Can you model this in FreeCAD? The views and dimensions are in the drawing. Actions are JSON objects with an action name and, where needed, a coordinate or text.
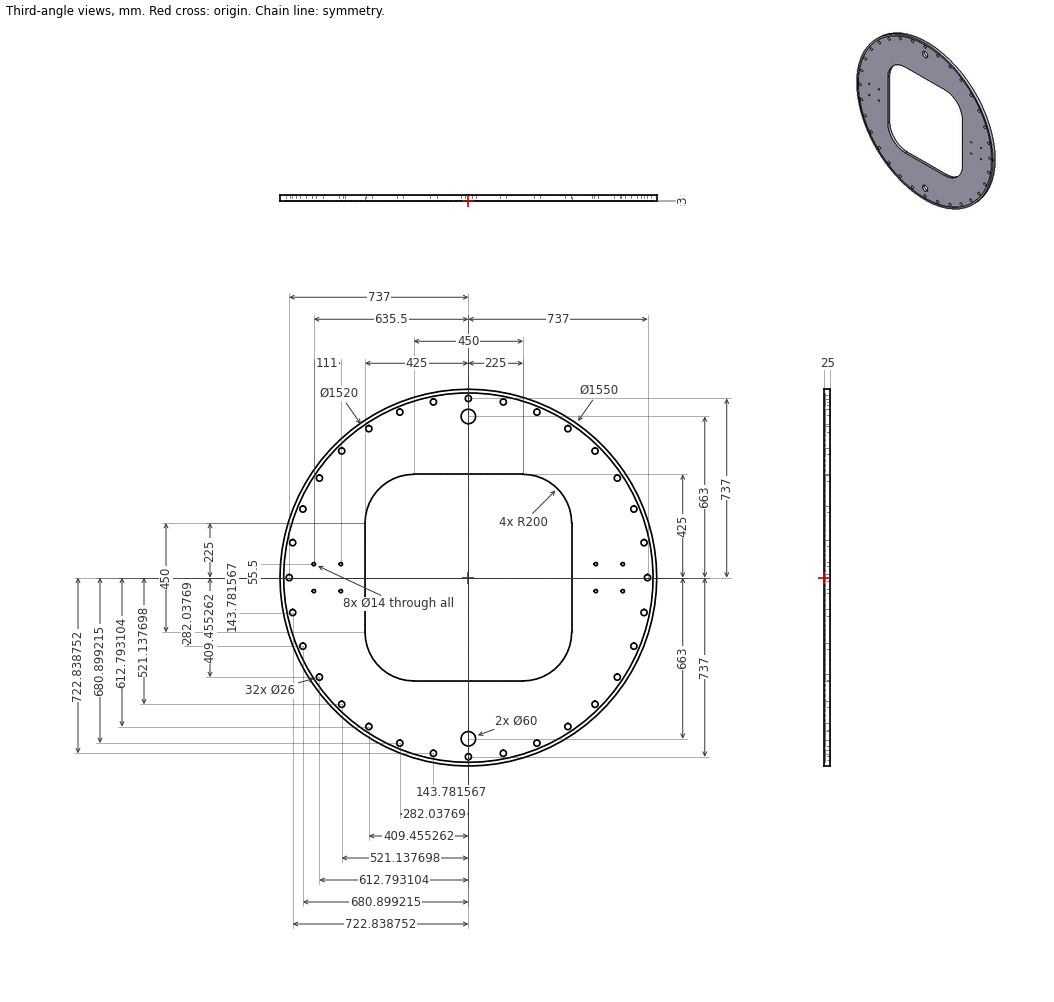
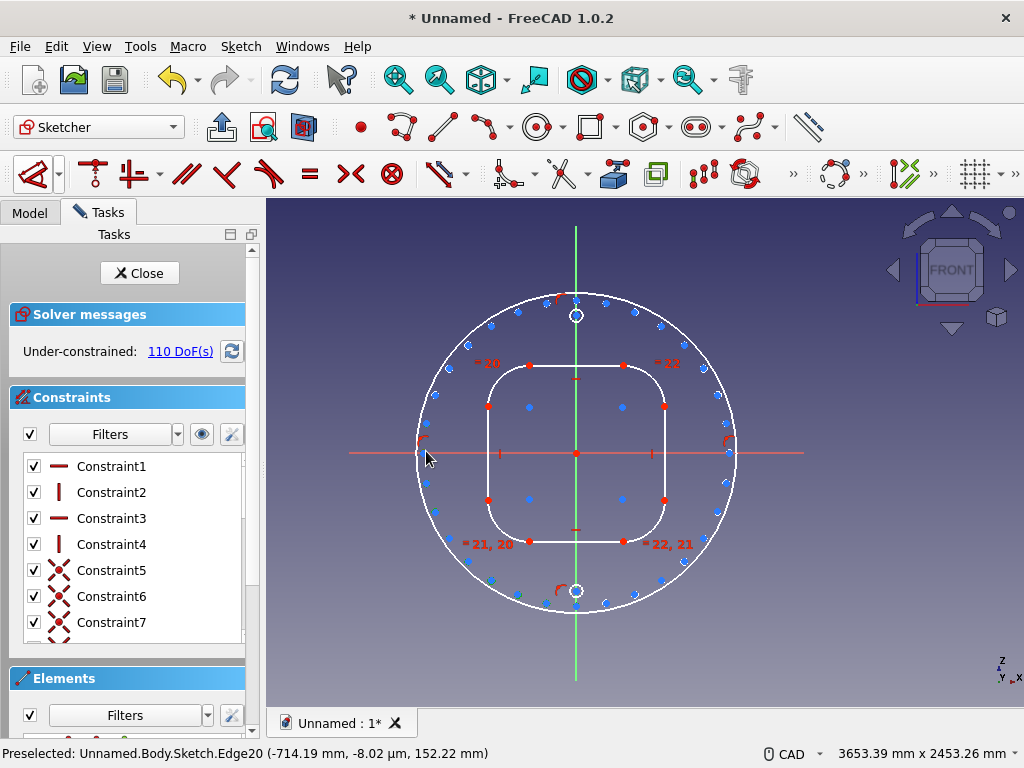
{"action": "scroll", "coordinate": [437, 393], "scroll_direction": "up", "scroll_amount": 8}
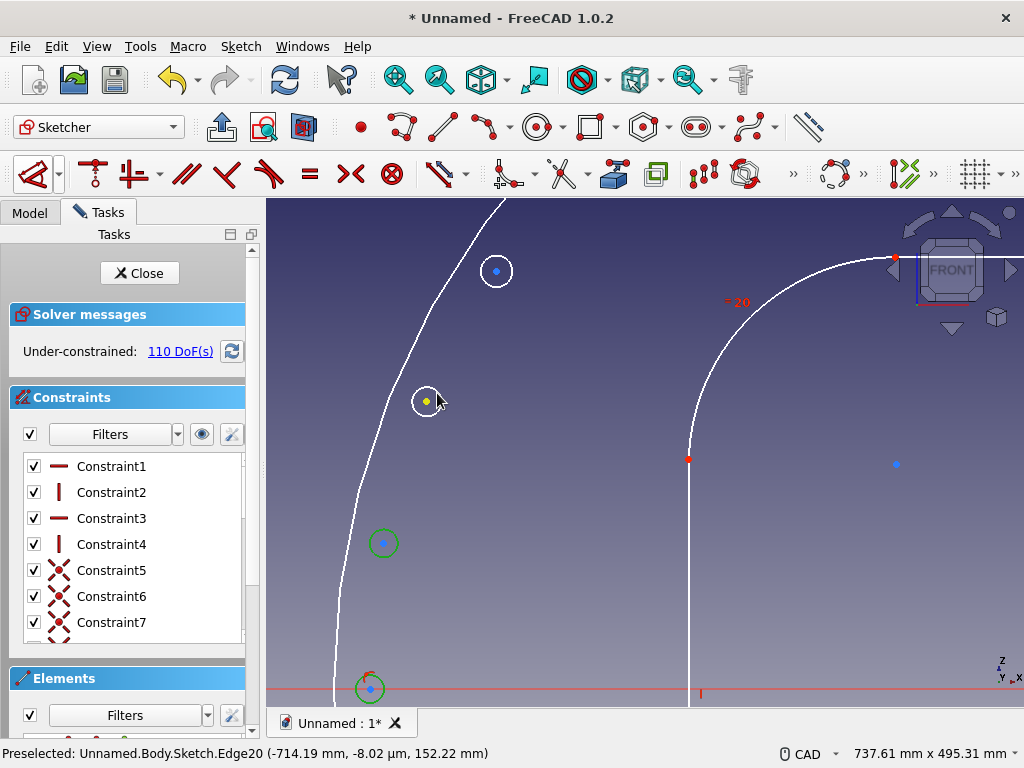
{"action": "left_click", "coordinate": [437, 391]}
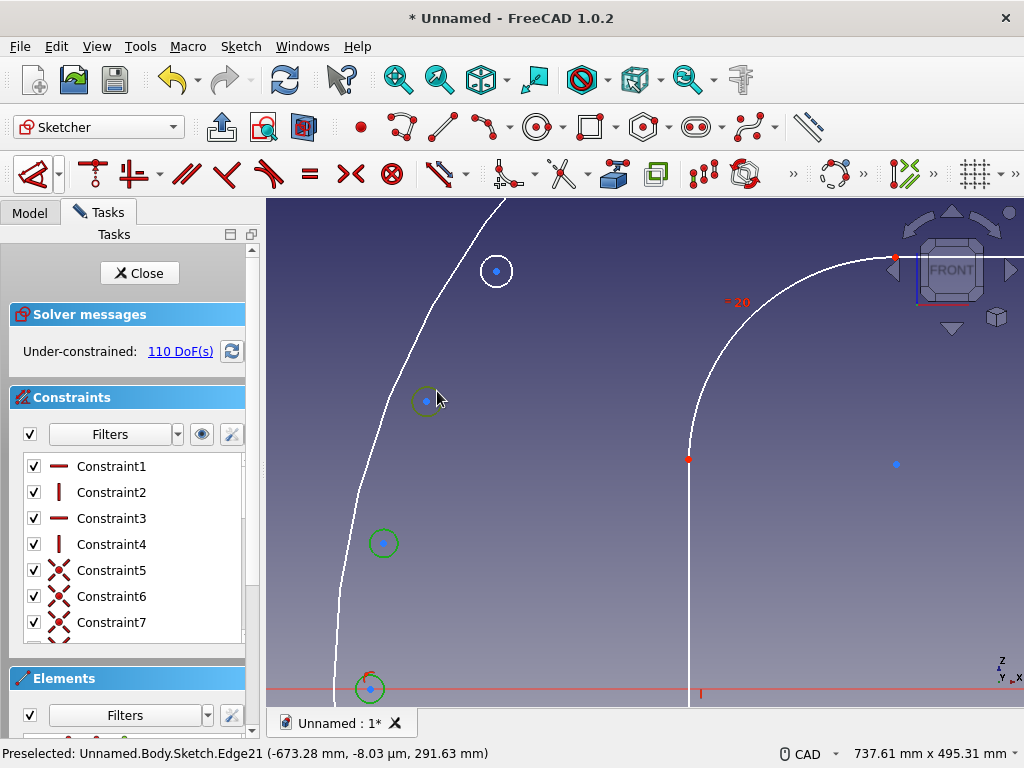
{"action": "left_click", "coordinate": [508, 260]}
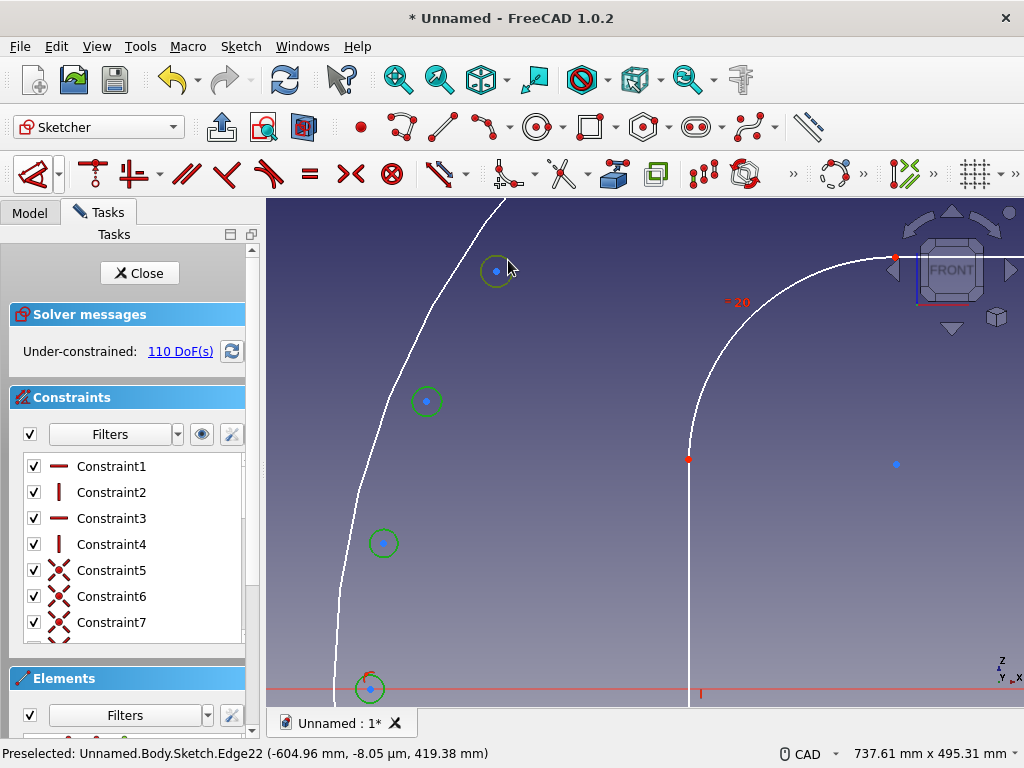
{"action": "scroll", "coordinate": [437, 393], "scroll_direction": "down", "scroll_amount": 8}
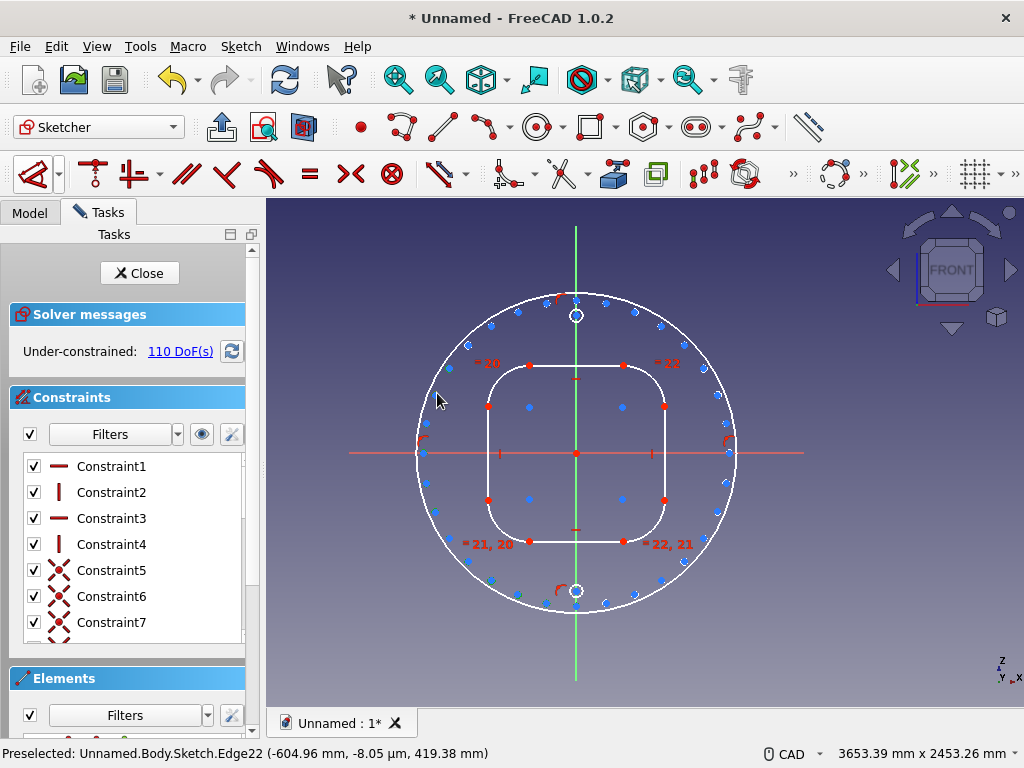
{"action": "scroll", "coordinate": [470, 343], "scroll_direction": "up", "scroll_amount": 8}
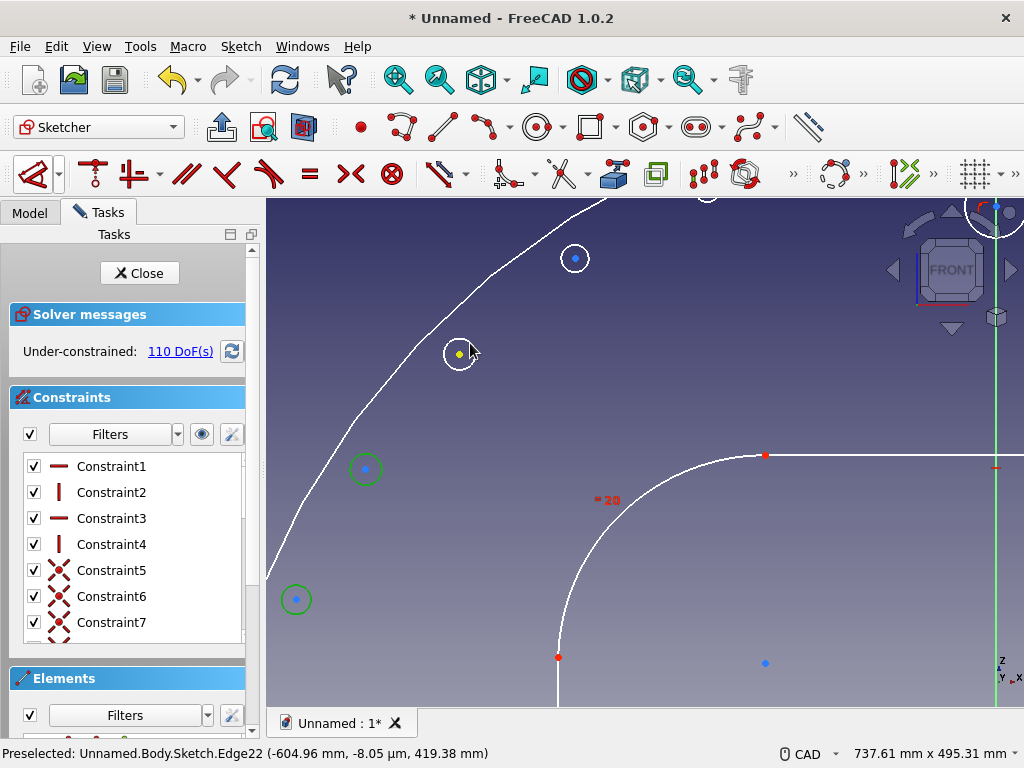
{"action": "left_click", "coordinate": [471, 343]}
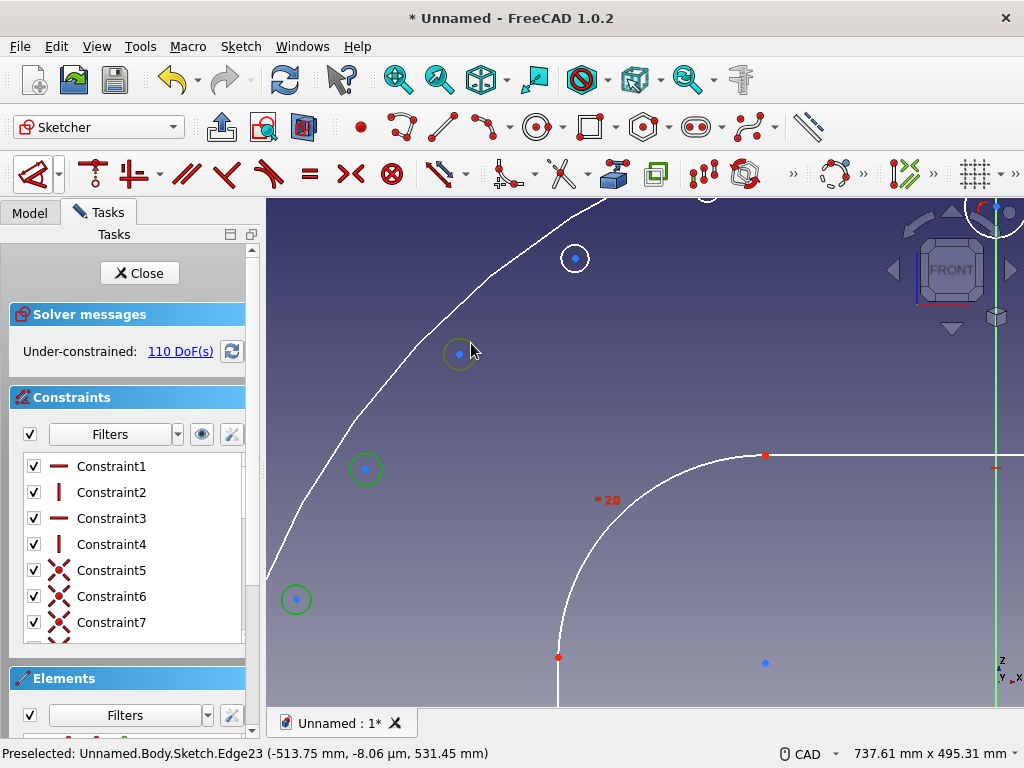
{"action": "left_click", "coordinate": [585, 249]}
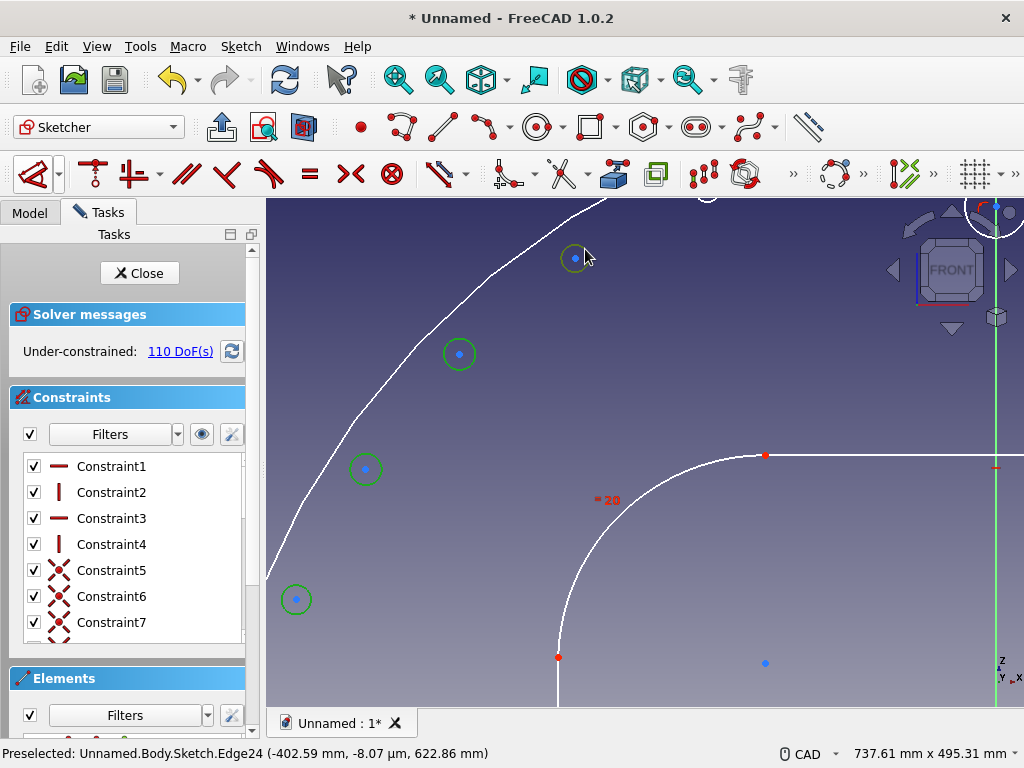
{"action": "scroll", "coordinate": [470, 343], "scroll_direction": "down", "scroll_amount": 8}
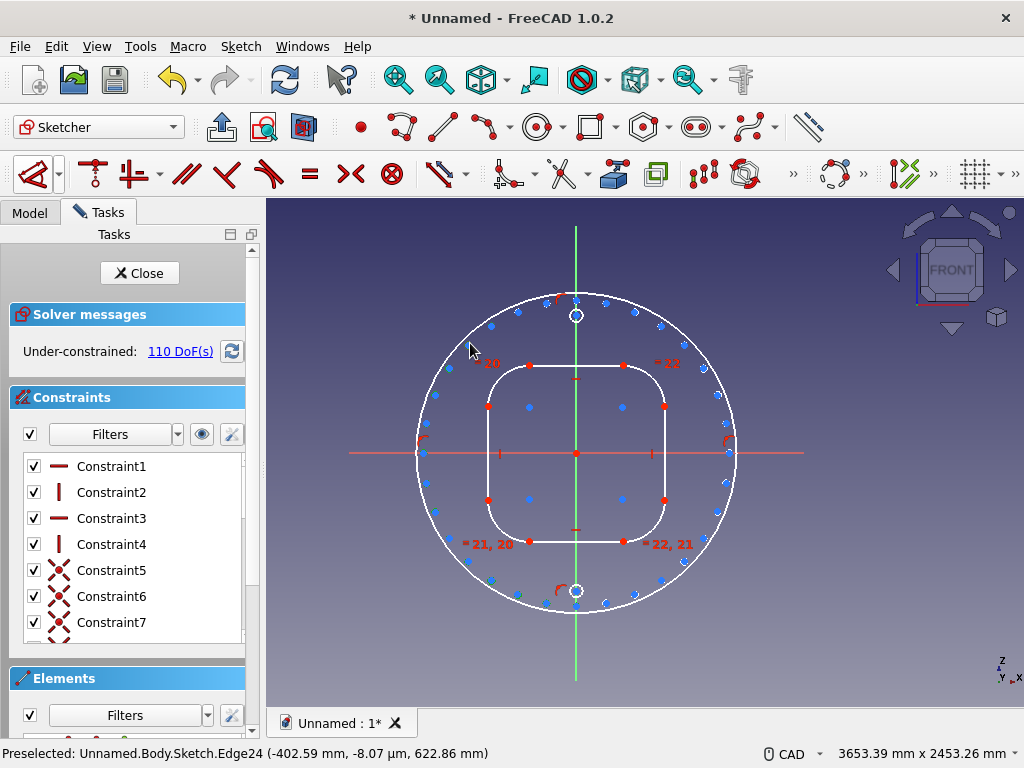
{"action": "scroll", "coordinate": [520, 310], "scroll_direction": "up", "scroll_amount": 9}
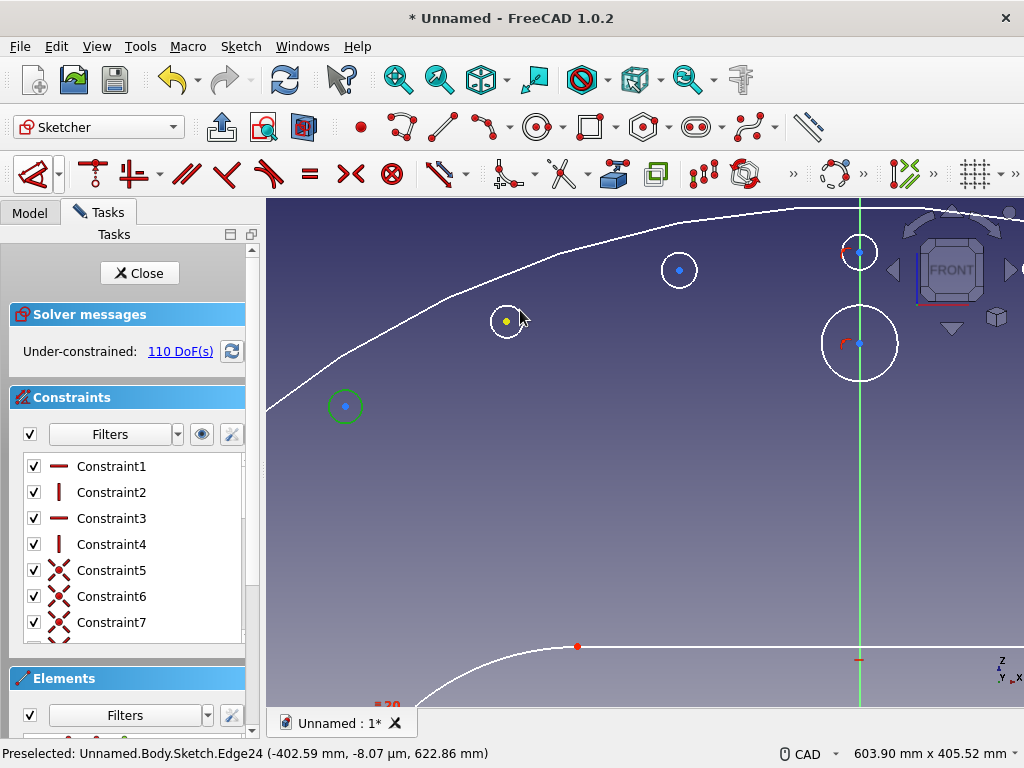
{"action": "left_click", "coordinate": [518, 310]}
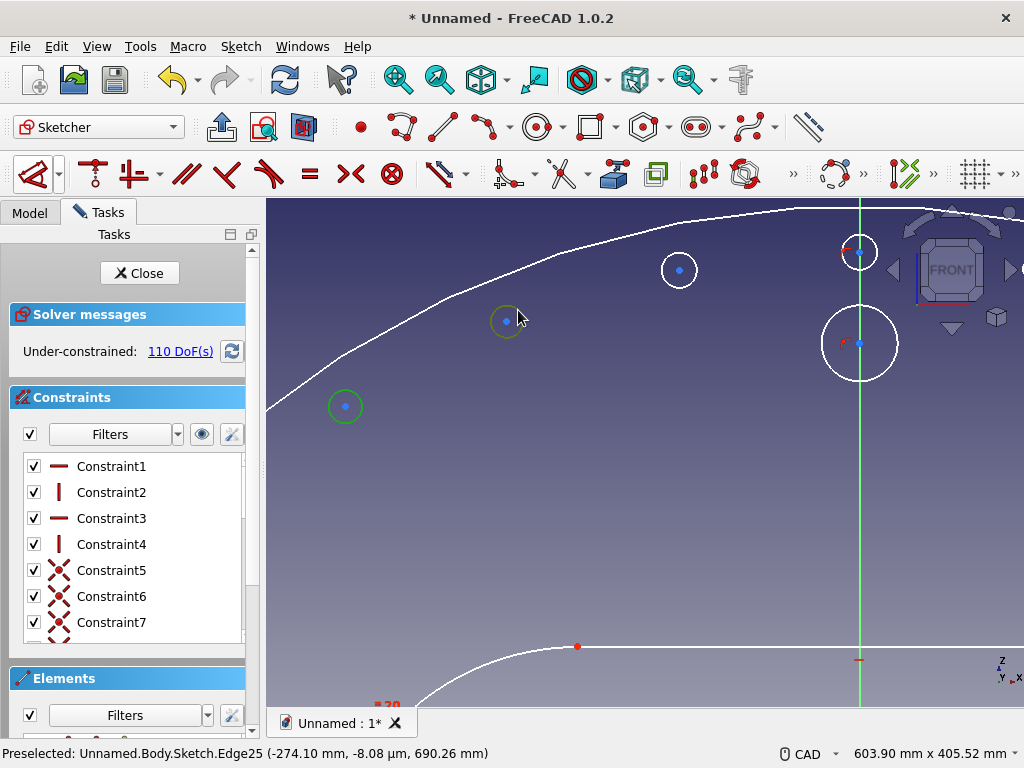
{"action": "left_click", "coordinate": [692, 258]}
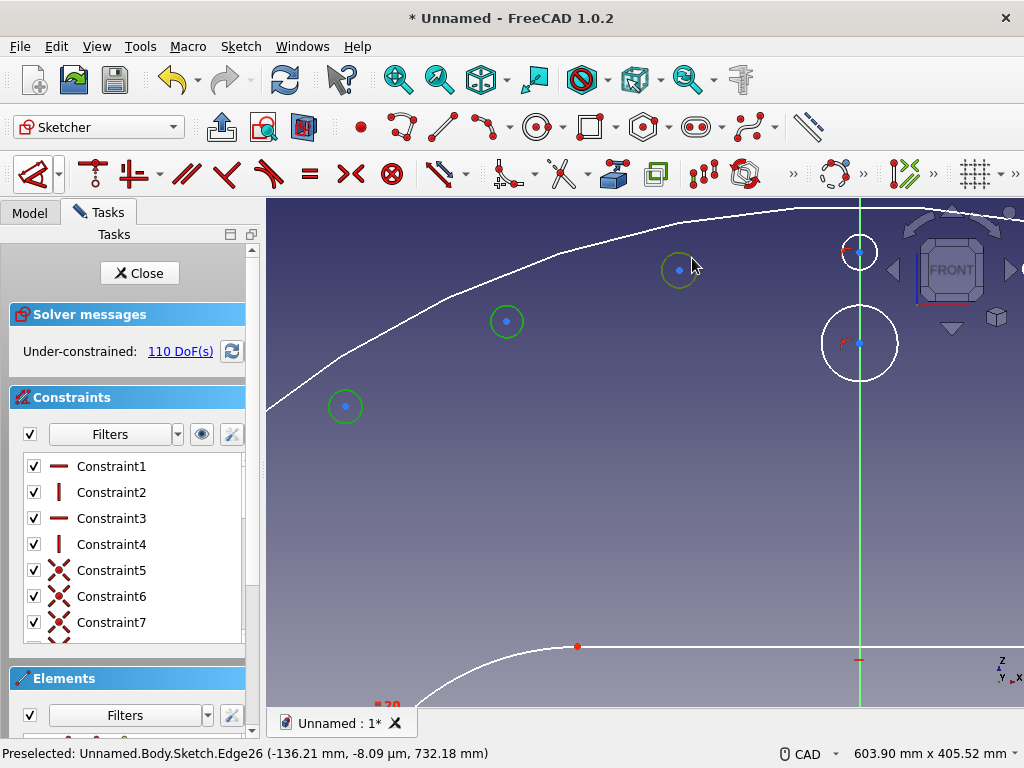
{"action": "scroll", "coordinate": [520, 310], "scroll_direction": "down", "scroll_amount": 9}